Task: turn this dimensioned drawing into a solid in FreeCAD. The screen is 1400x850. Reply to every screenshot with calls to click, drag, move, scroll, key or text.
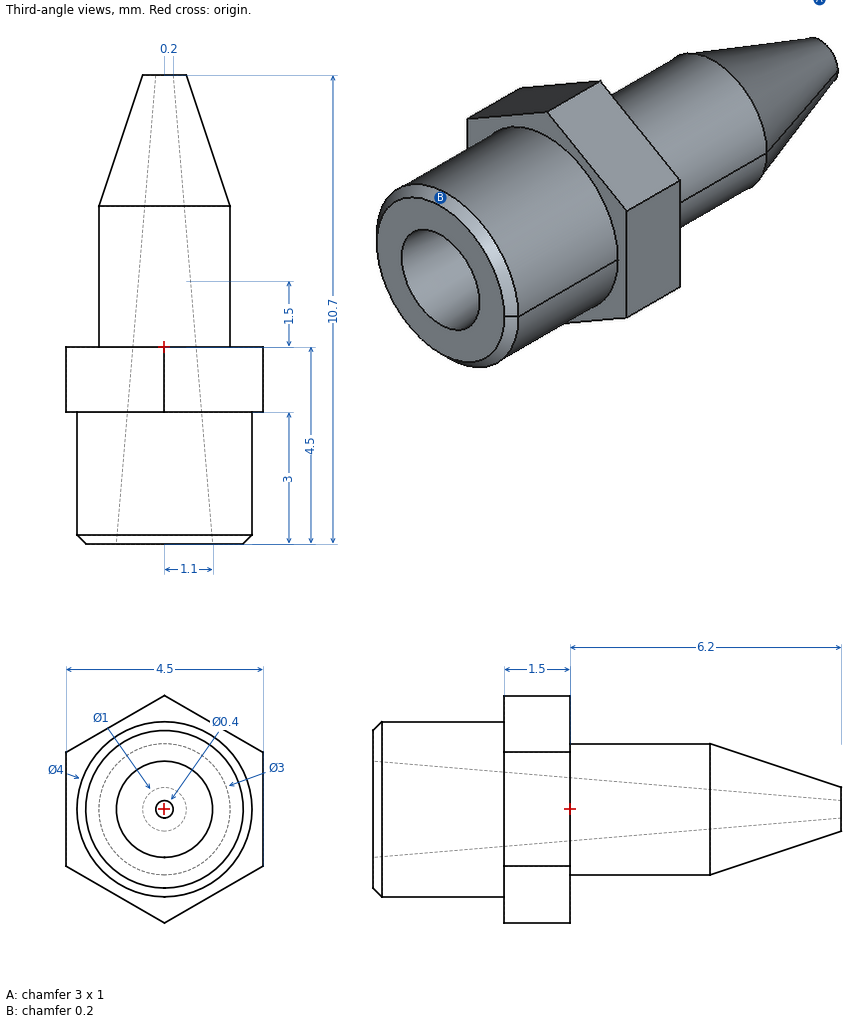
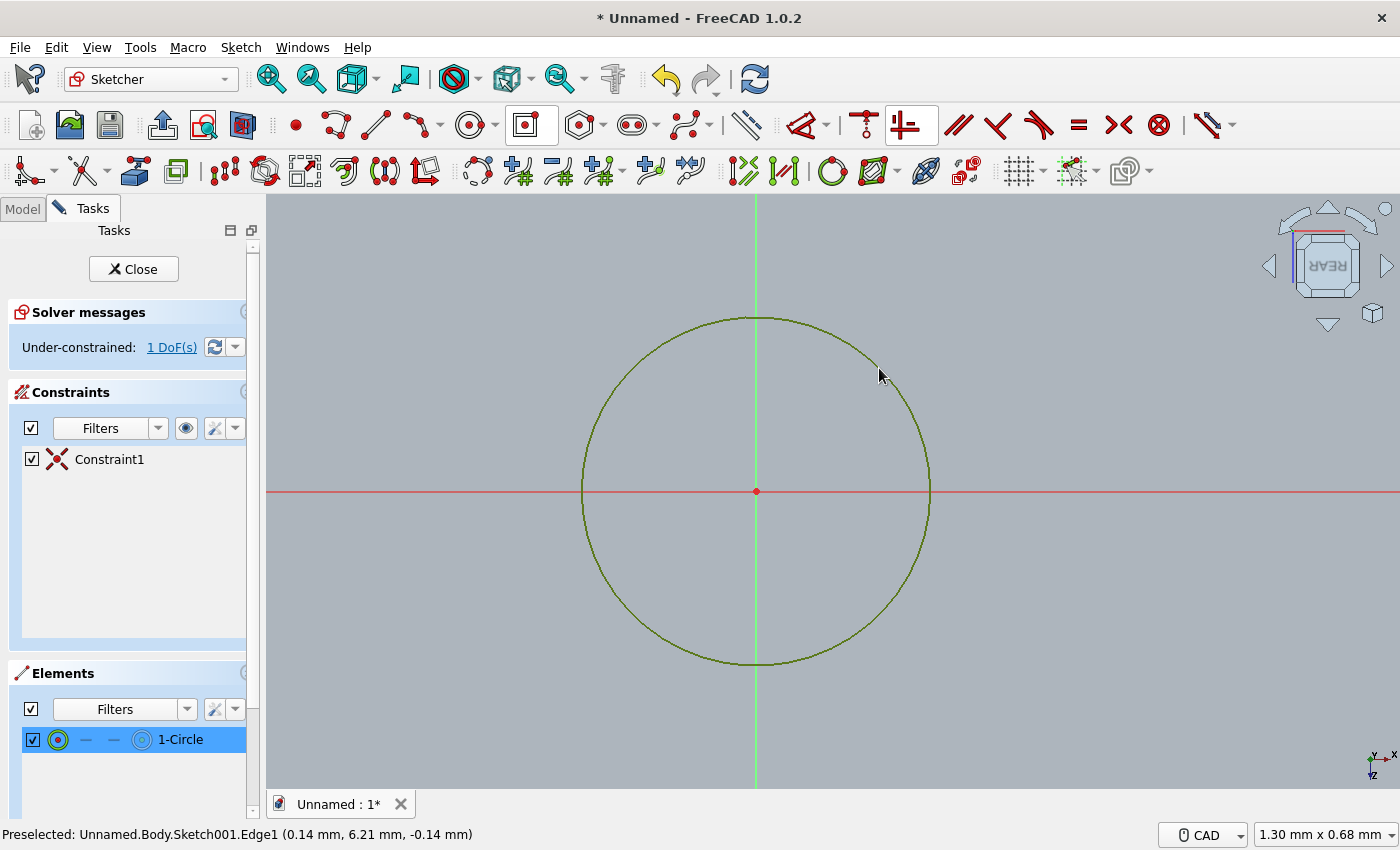
key(k)
key(o)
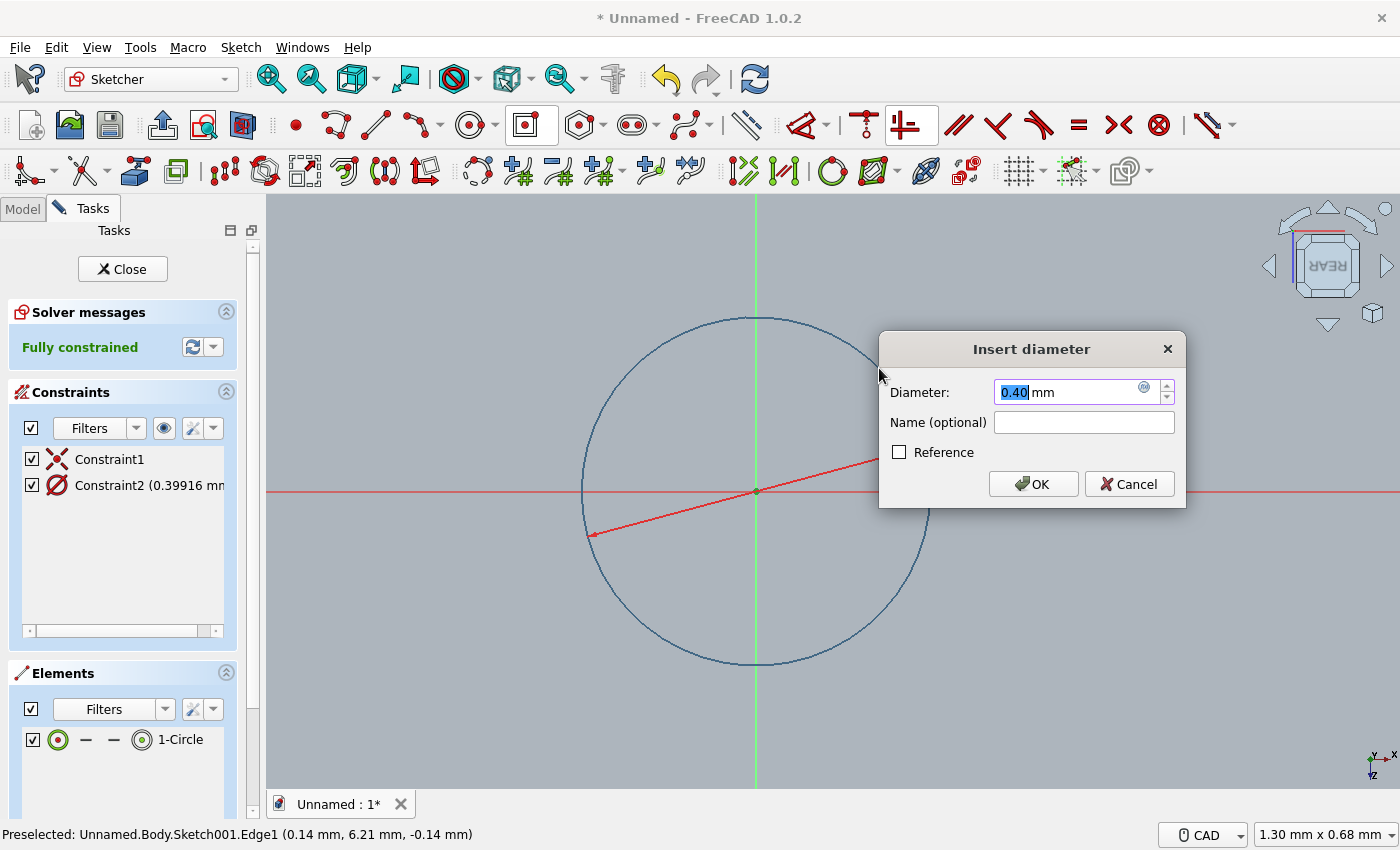
text(0.4)
key(Return)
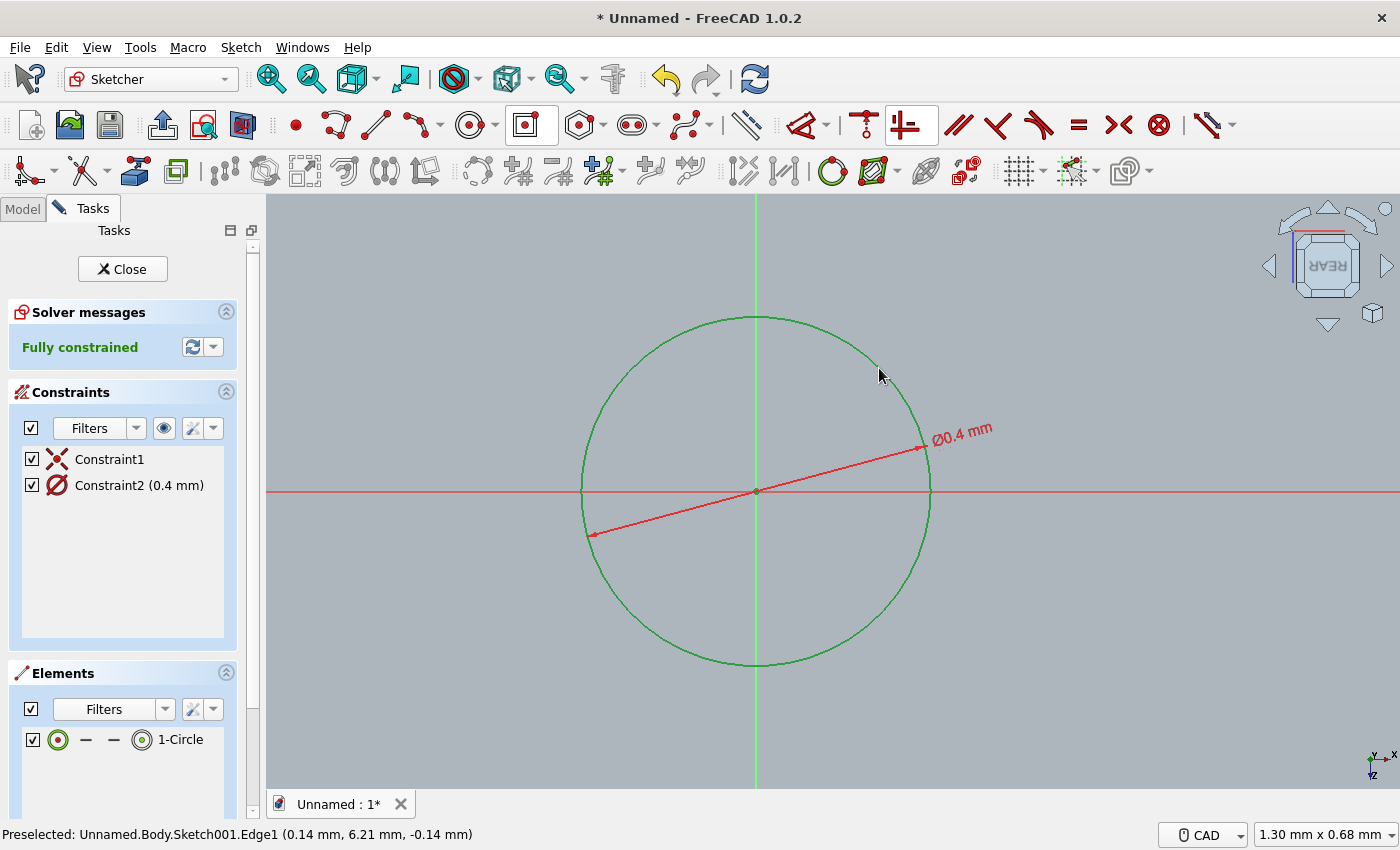
click(123, 269)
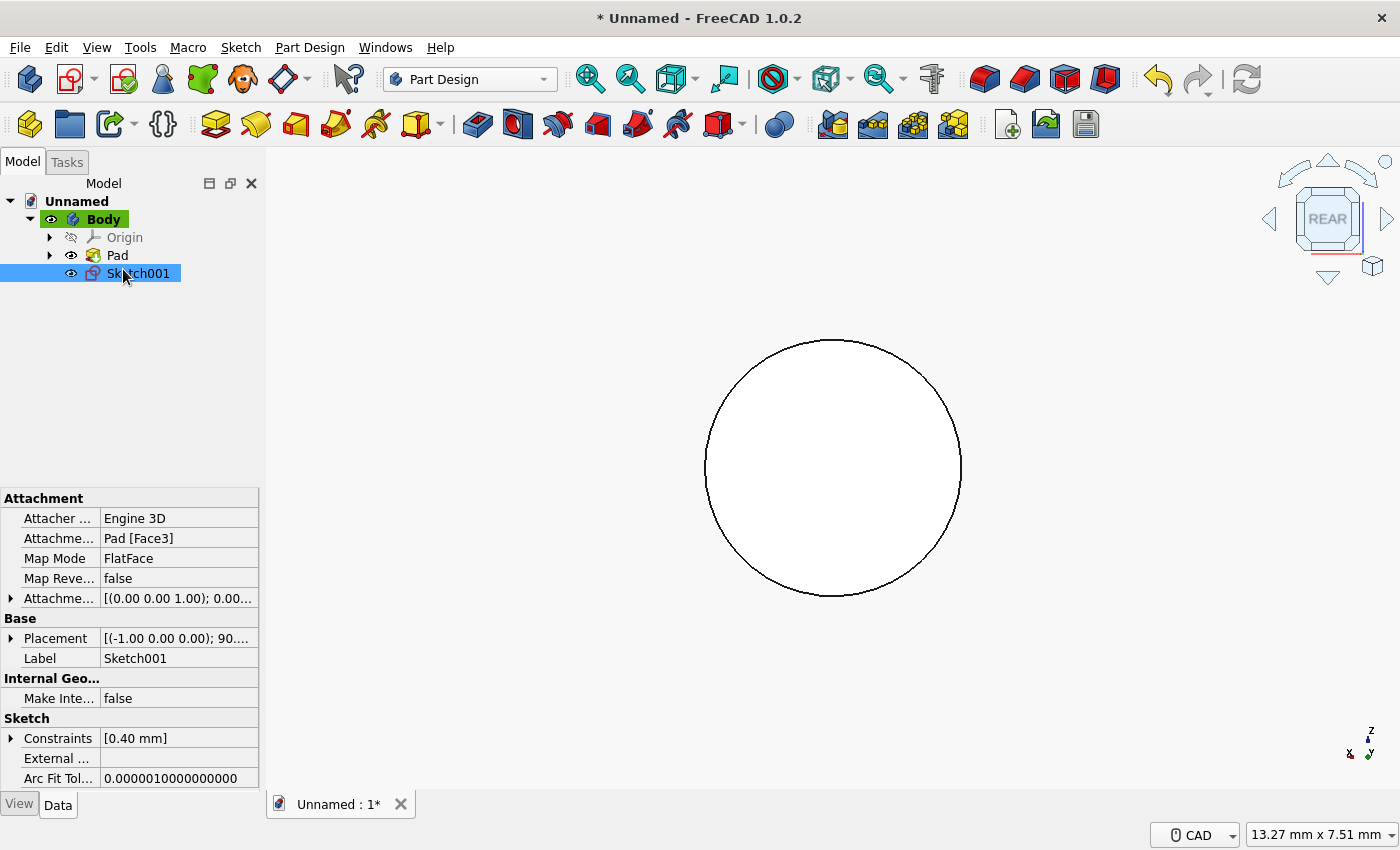
click(478, 124)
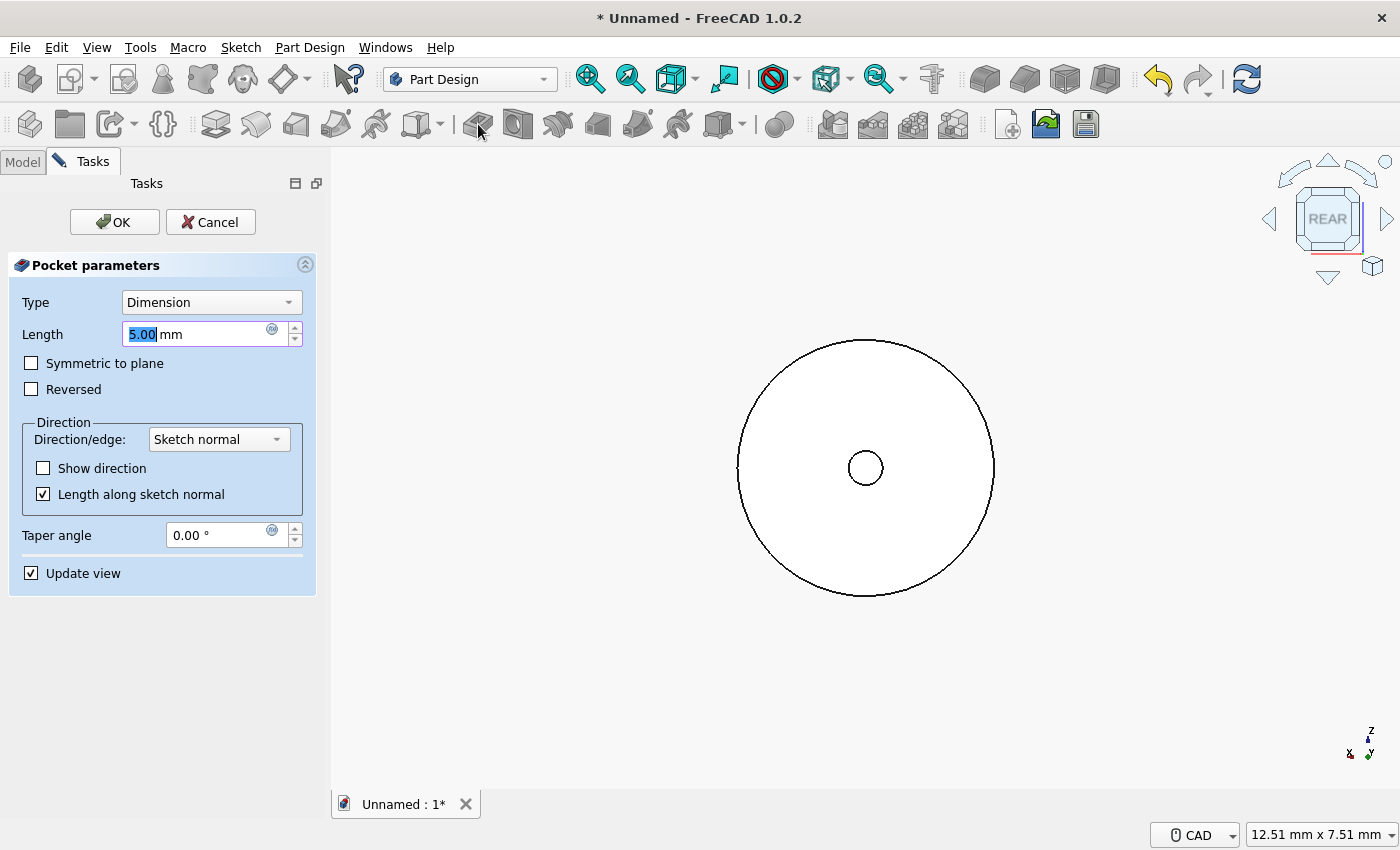
click(212, 302)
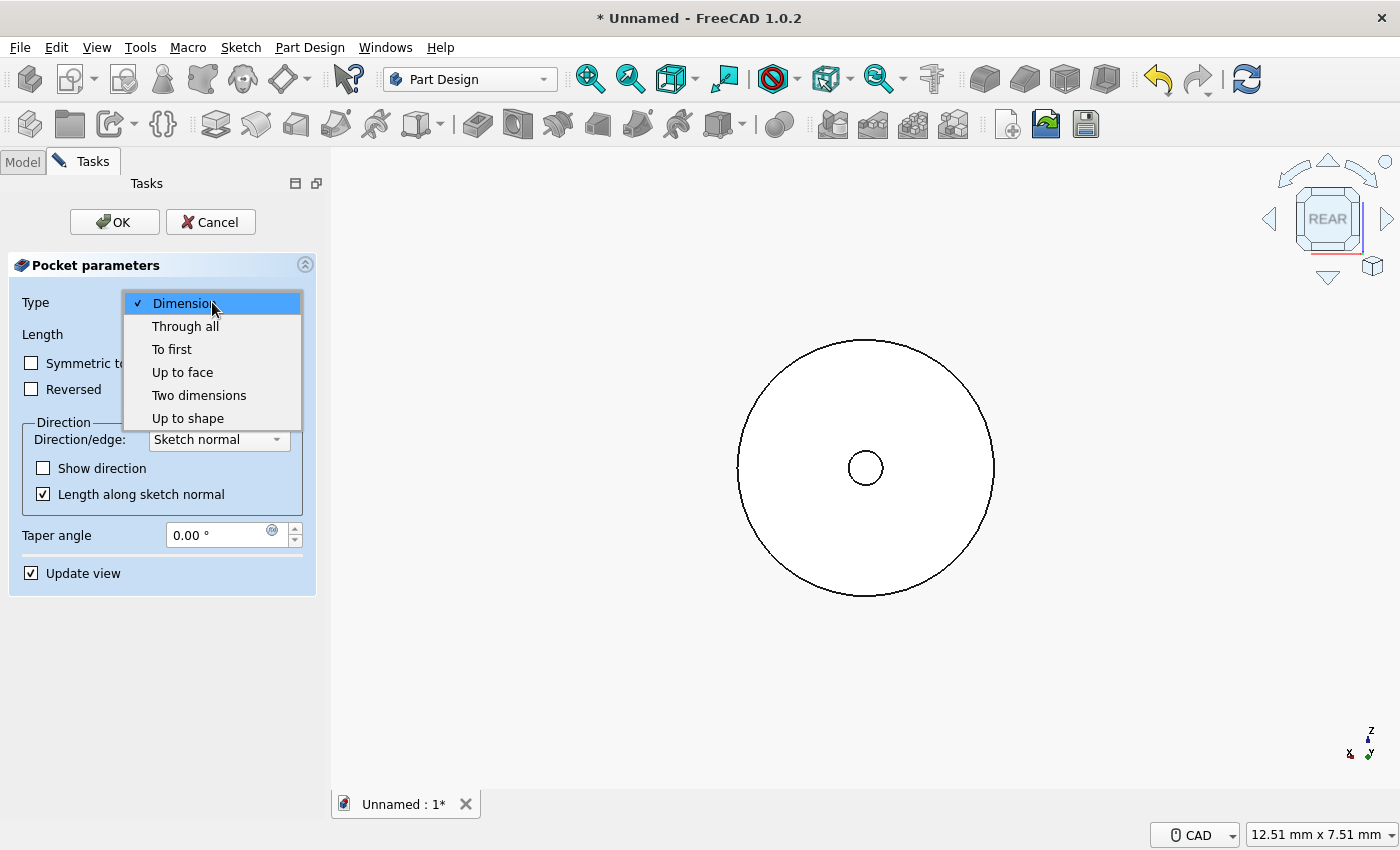
click(212, 326)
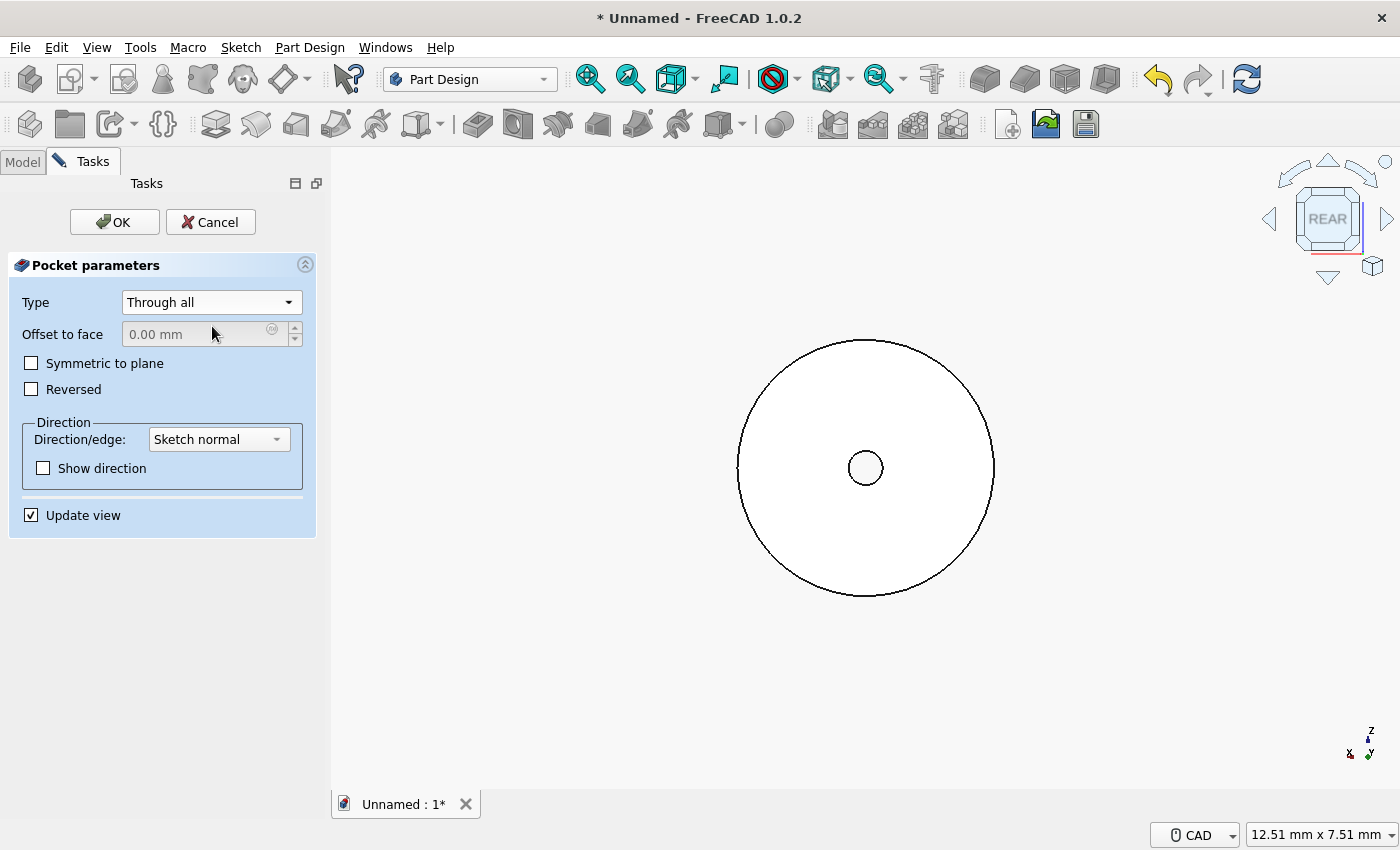
click(115, 222)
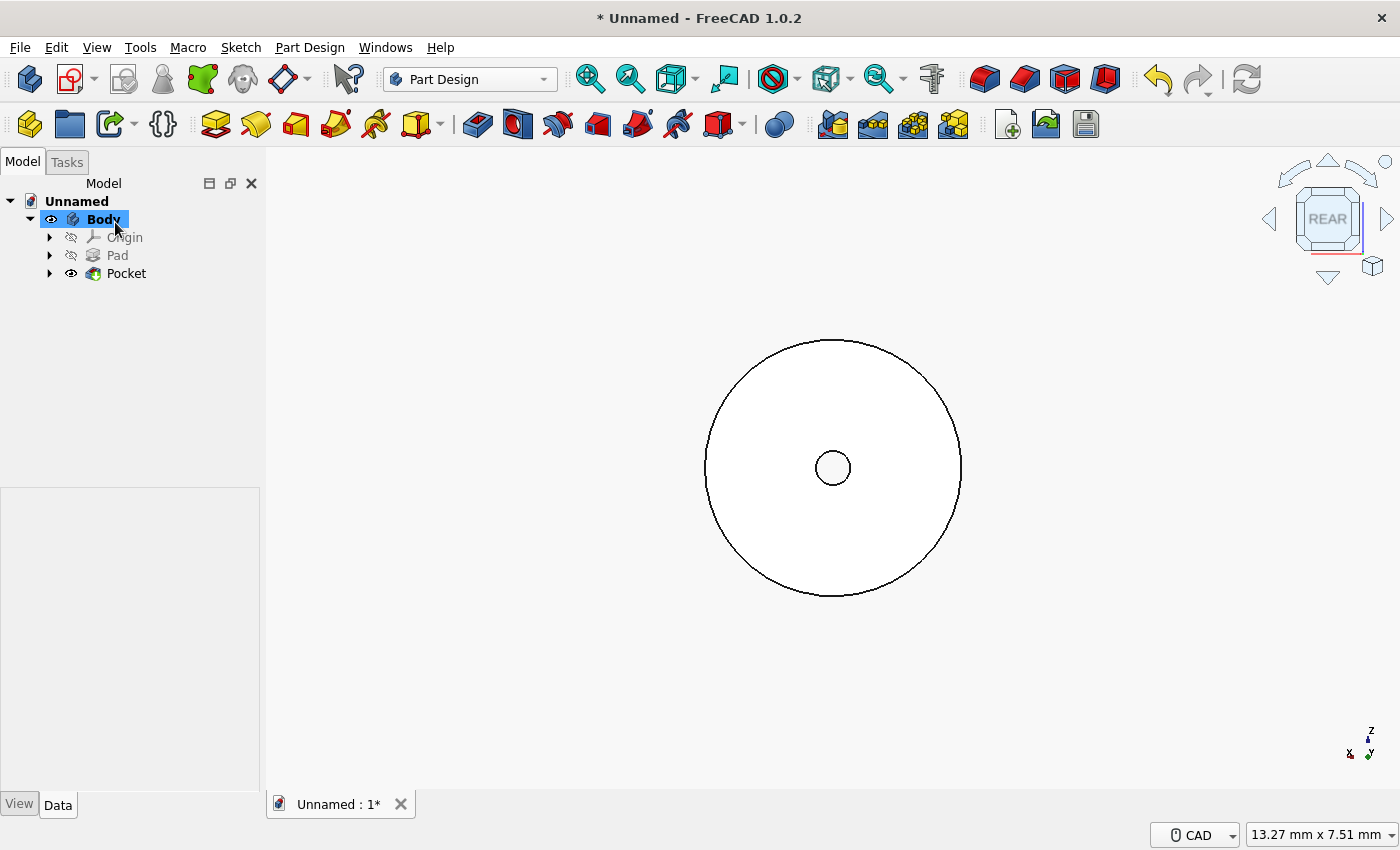
click(592, 80)